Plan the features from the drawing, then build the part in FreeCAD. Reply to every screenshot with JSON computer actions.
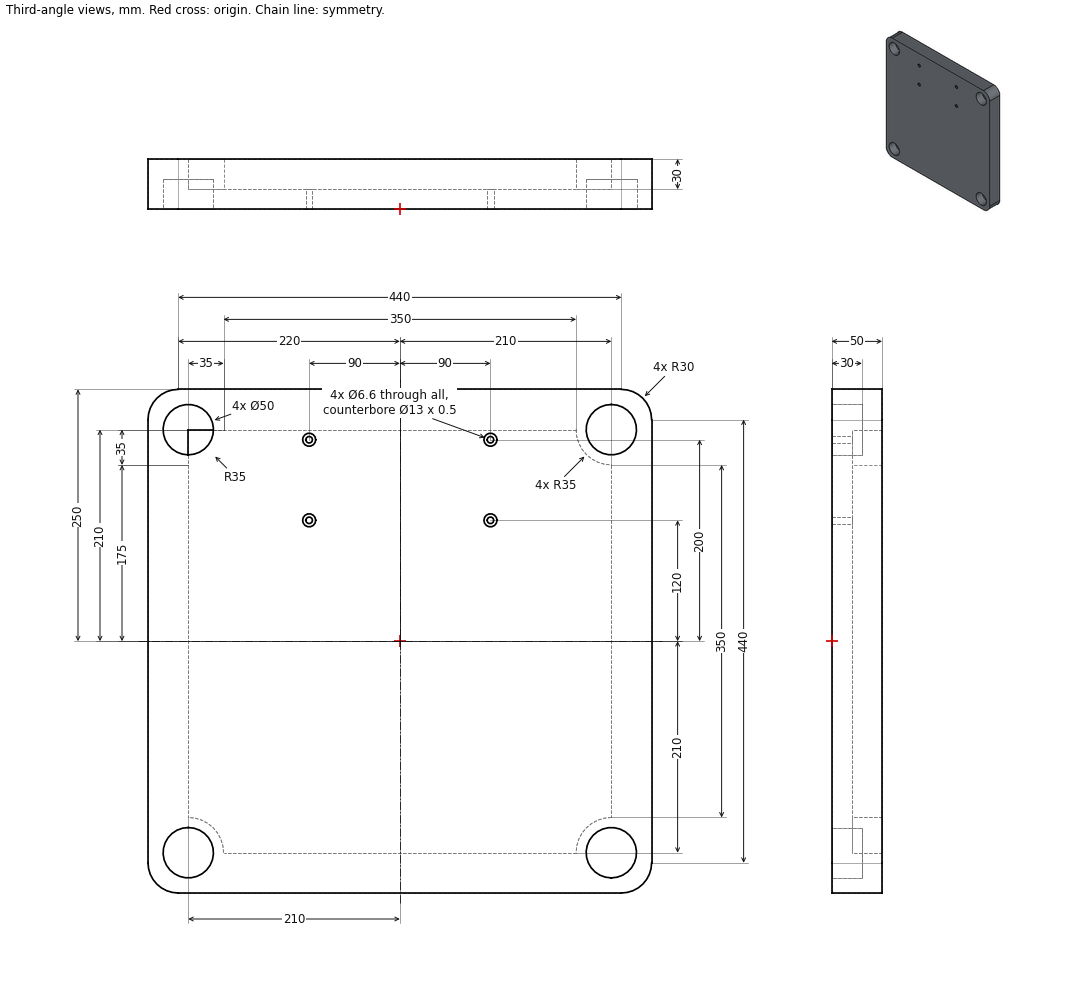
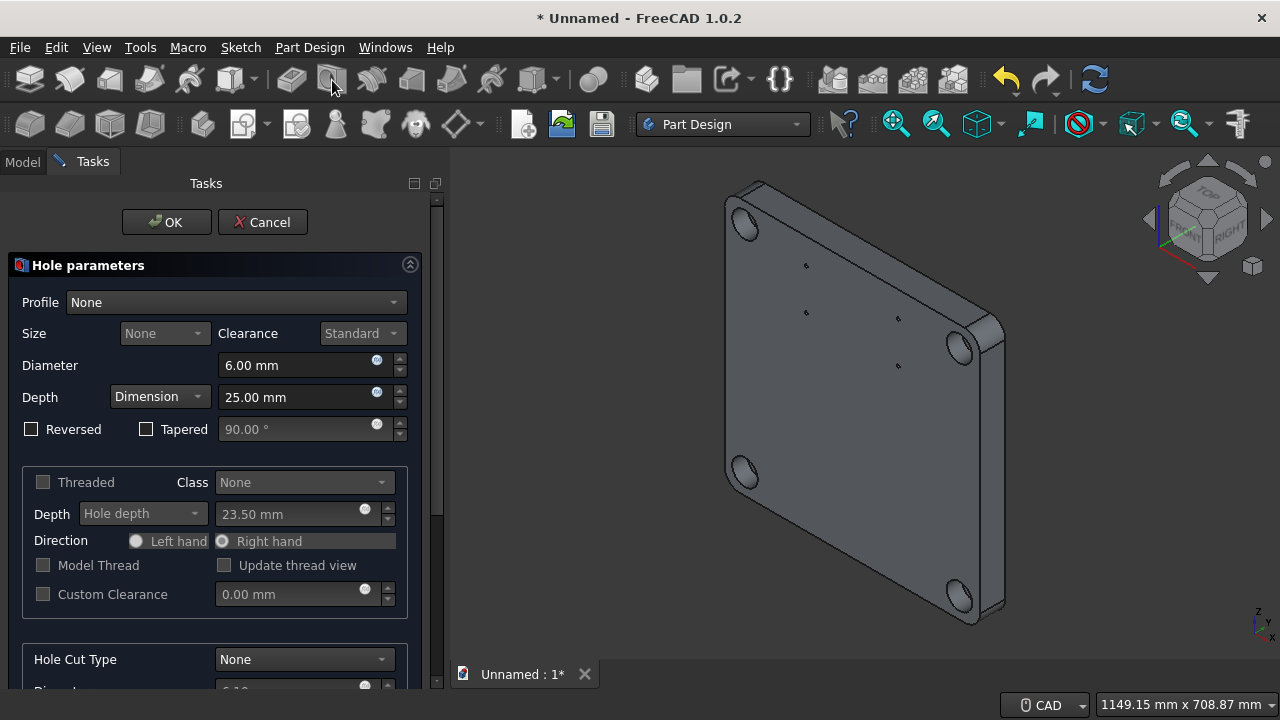
{"action": "triple_click", "coordinate": [305, 365]}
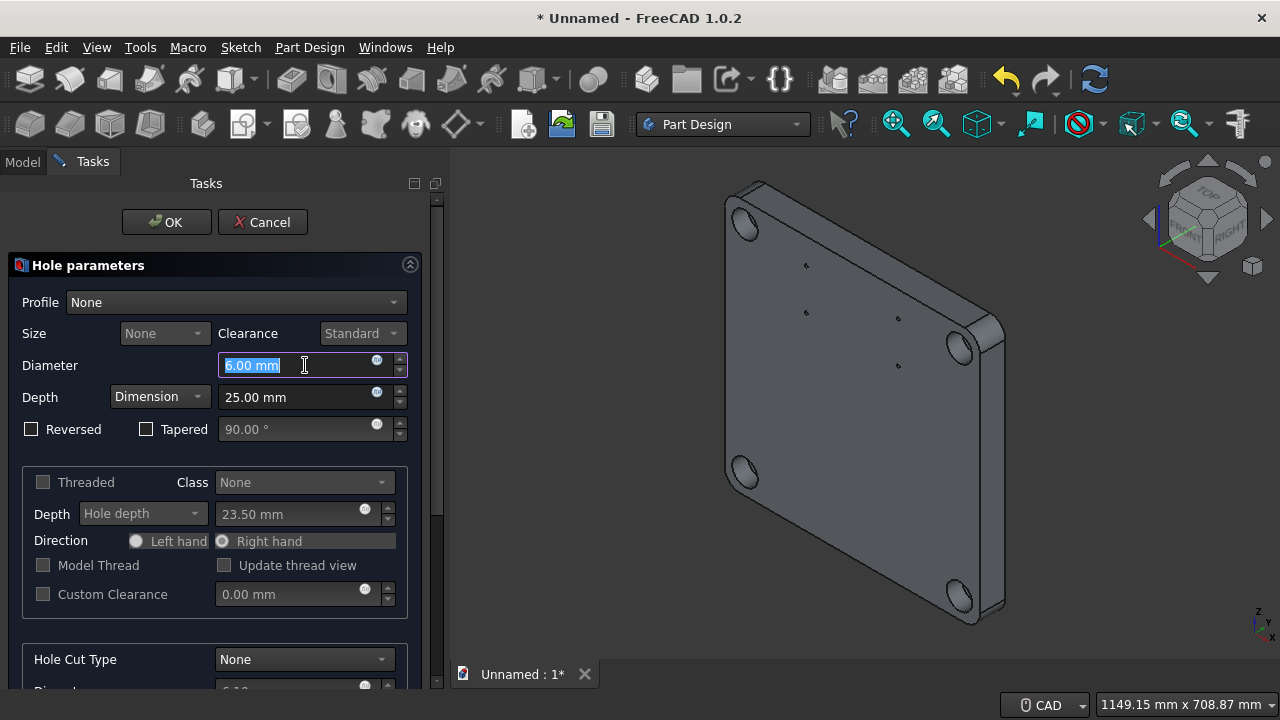
{"action": "type", "text": "6.6"}
{"action": "key", "text": "Tab"}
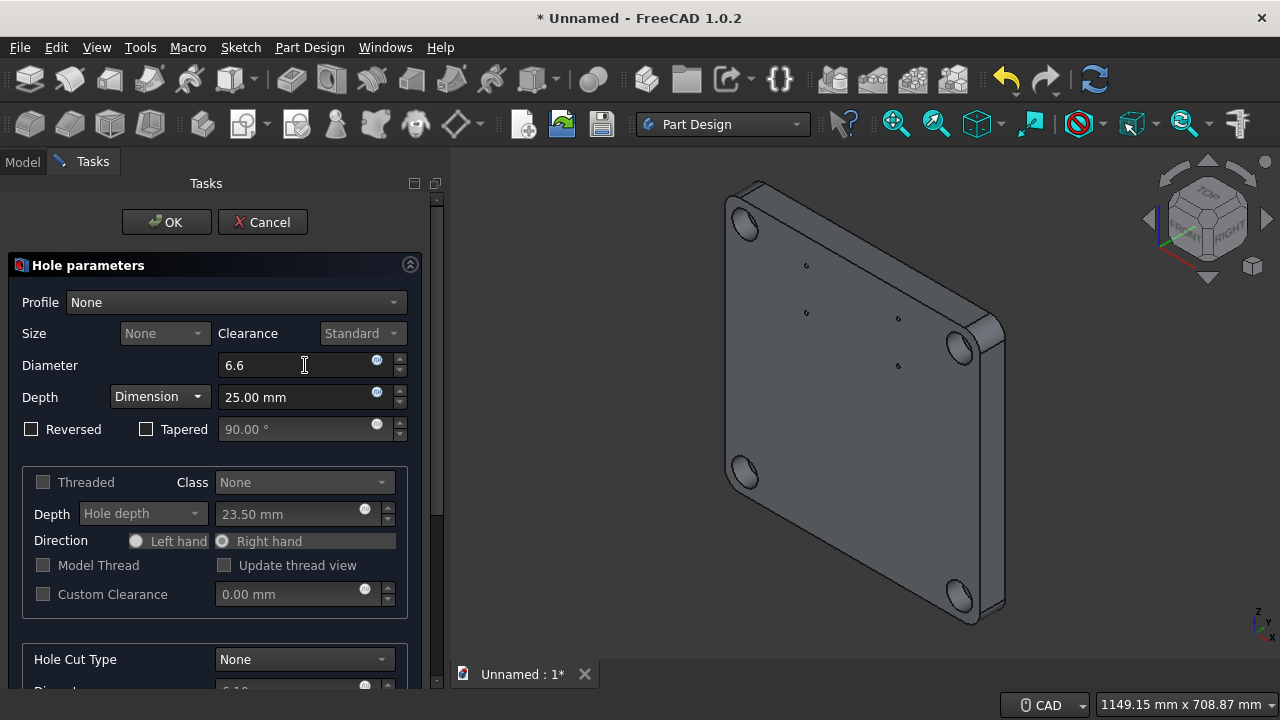
{"action": "left_click", "coordinate": [161, 396]}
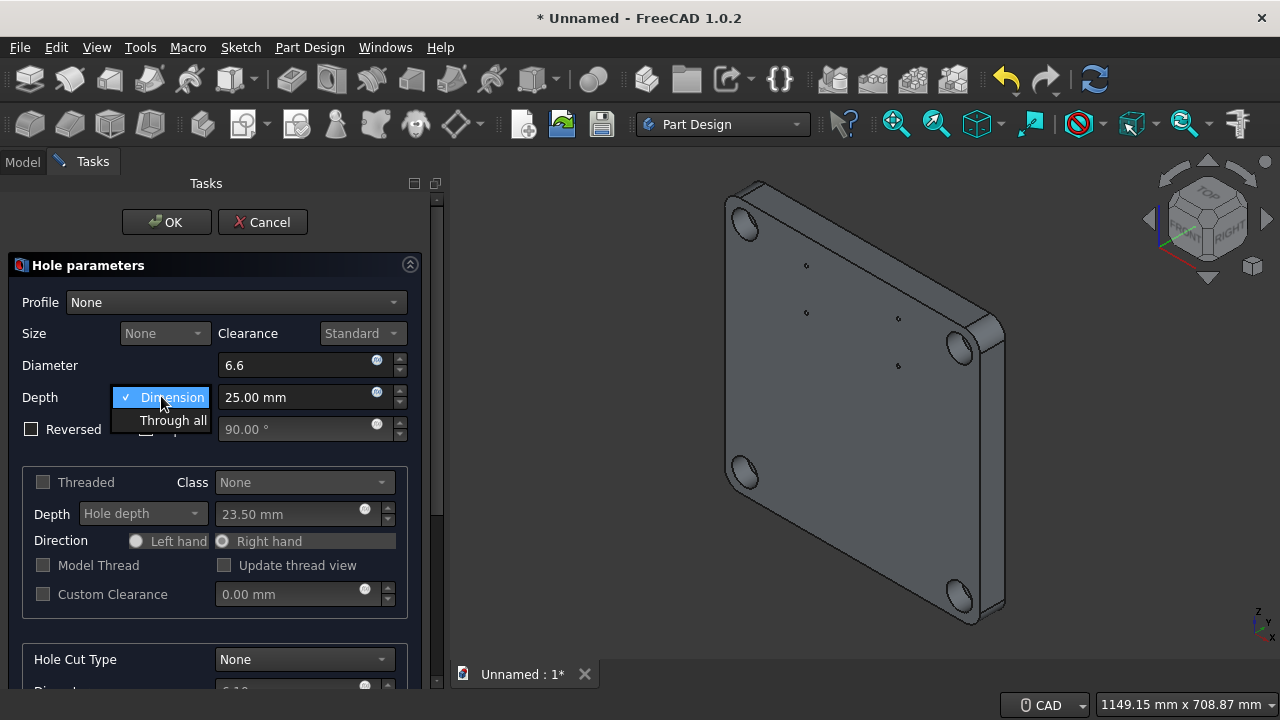
{"action": "left_click", "coordinate": [160, 420]}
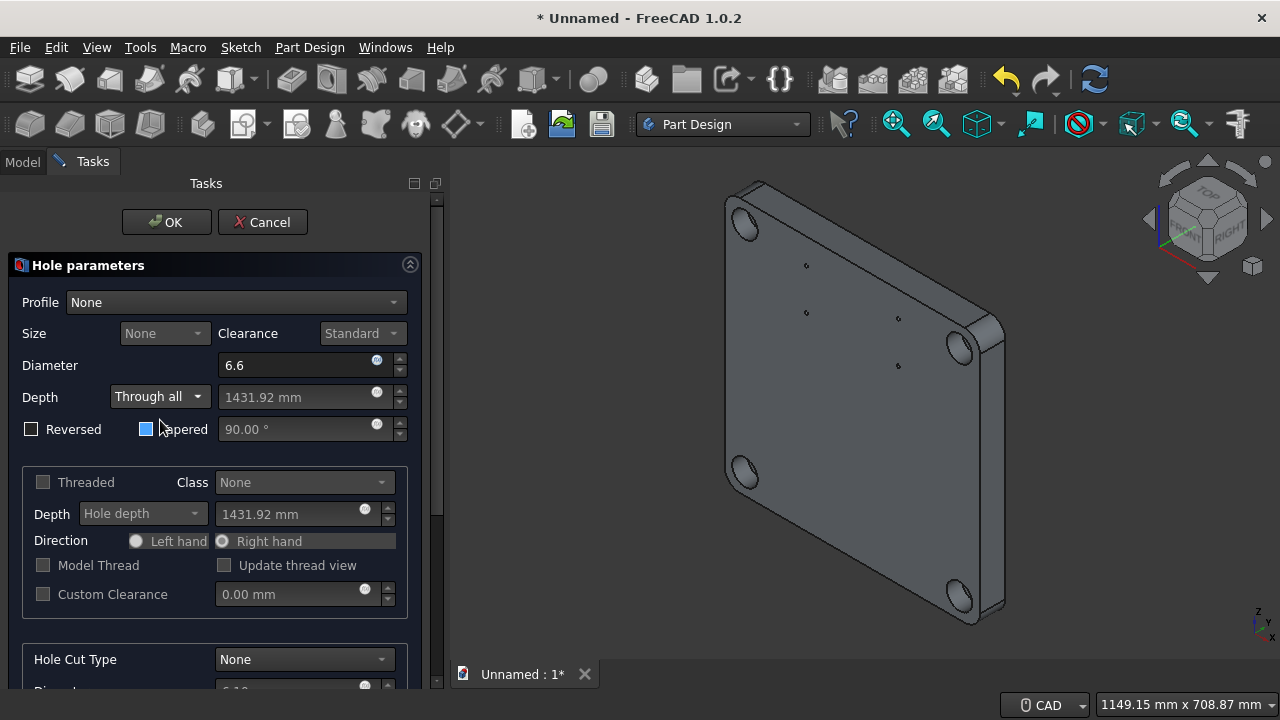
{"action": "left_click", "coordinate": [306, 660]}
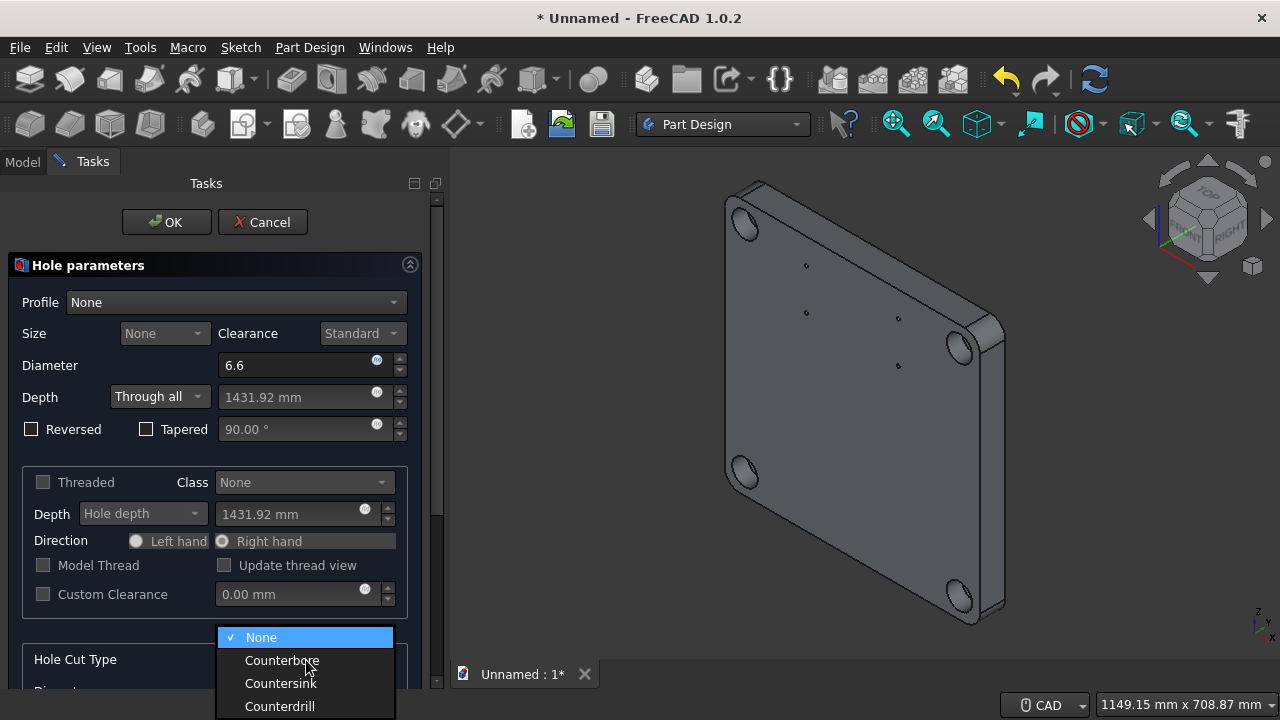
{"action": "left_click", "coordinate": [304, 660]}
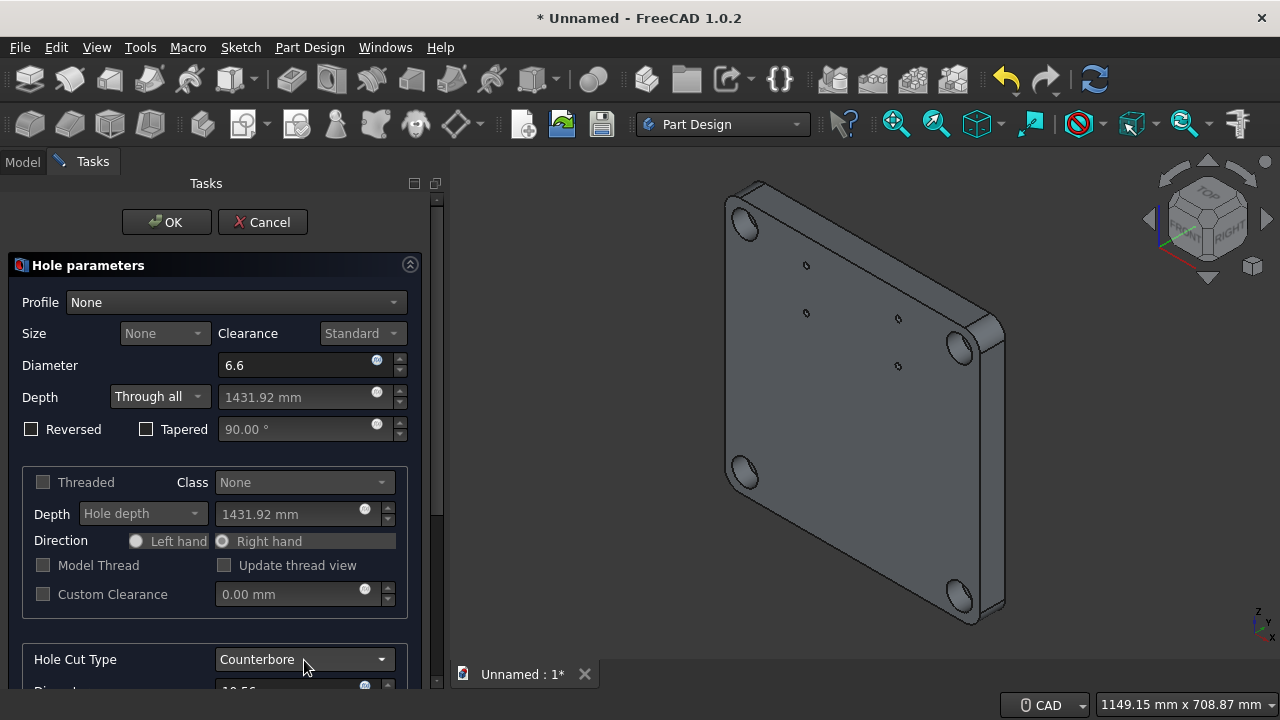
{"action": "scroll", "coordinate": [437, 440], "scroll_direction": "down", "scroll_amount": 2}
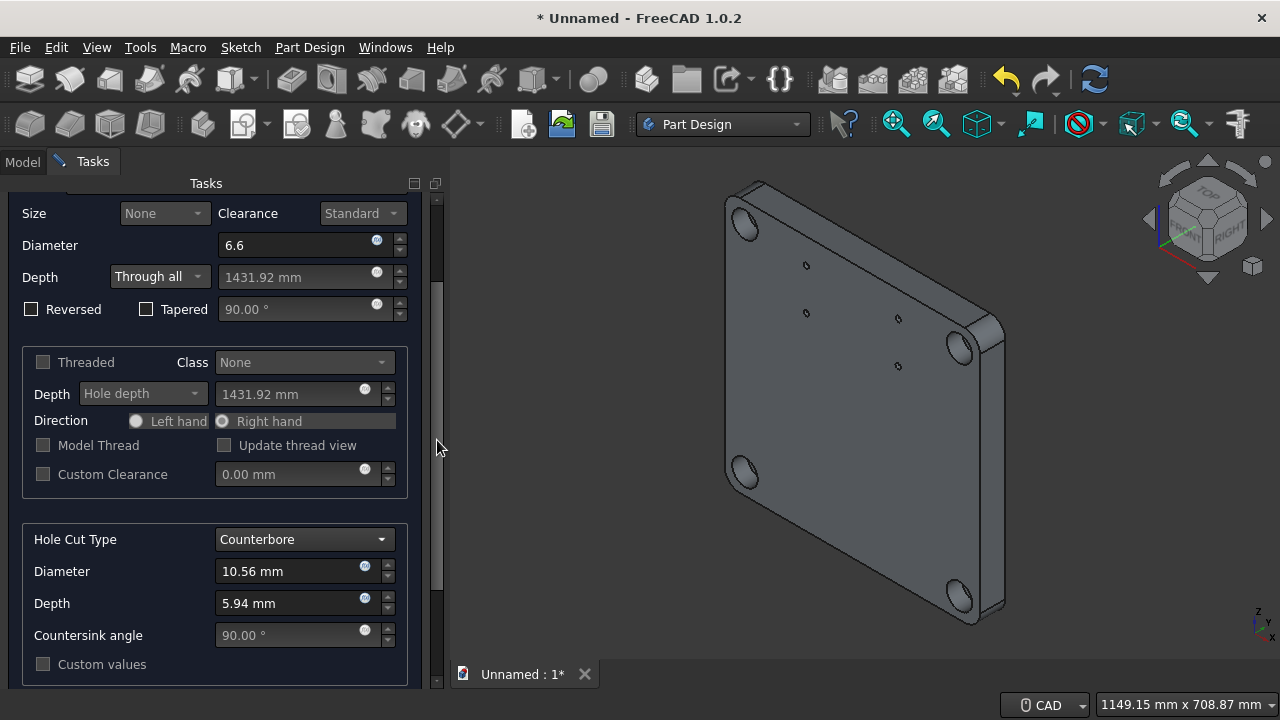
{"action": "triple_click", "coordinate": [298, 571]}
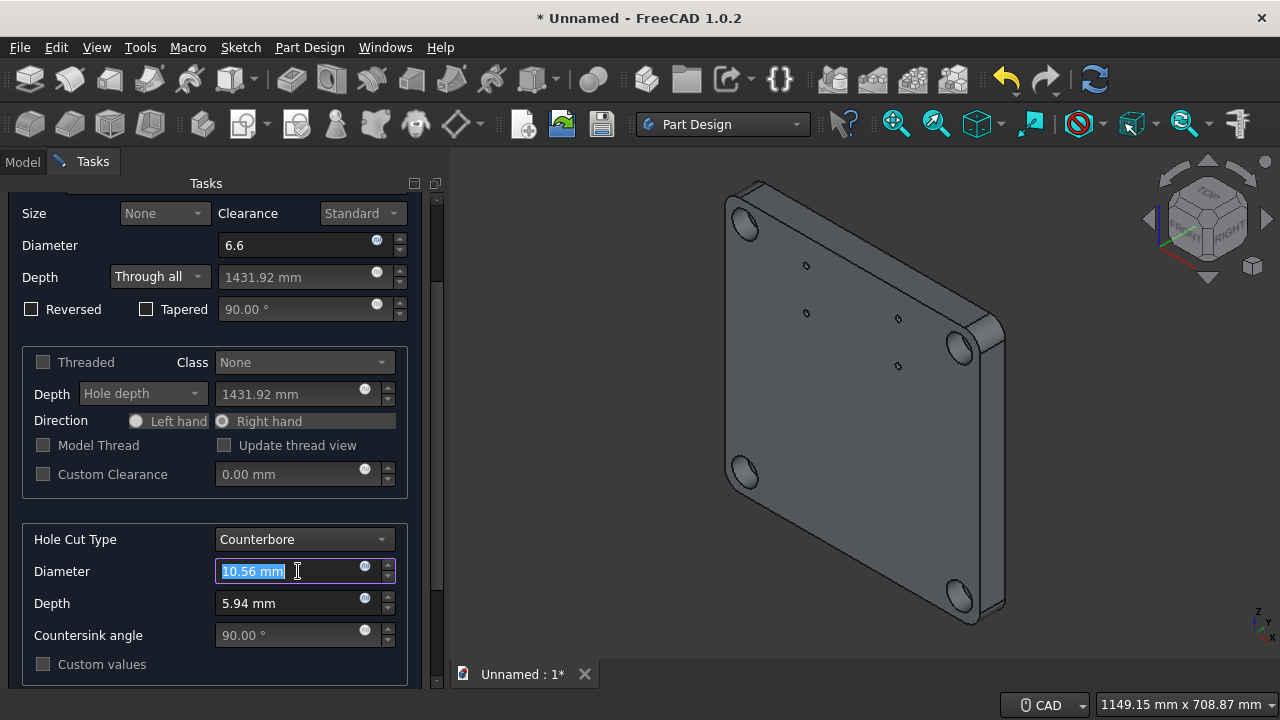
{"action": "type", "text": "13"}
{"action": "key", "text": "Tab"}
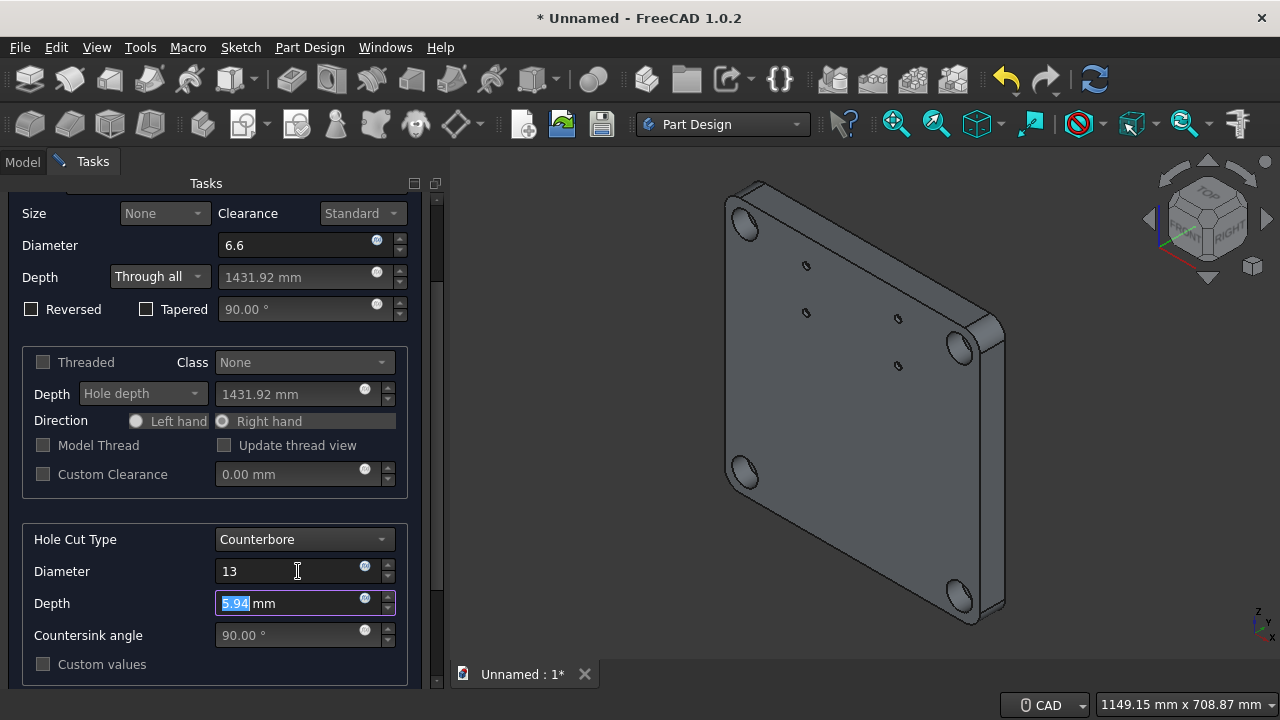
{"action": "type", "text": "0.5"}
{"action": "key", "text": "Tab"}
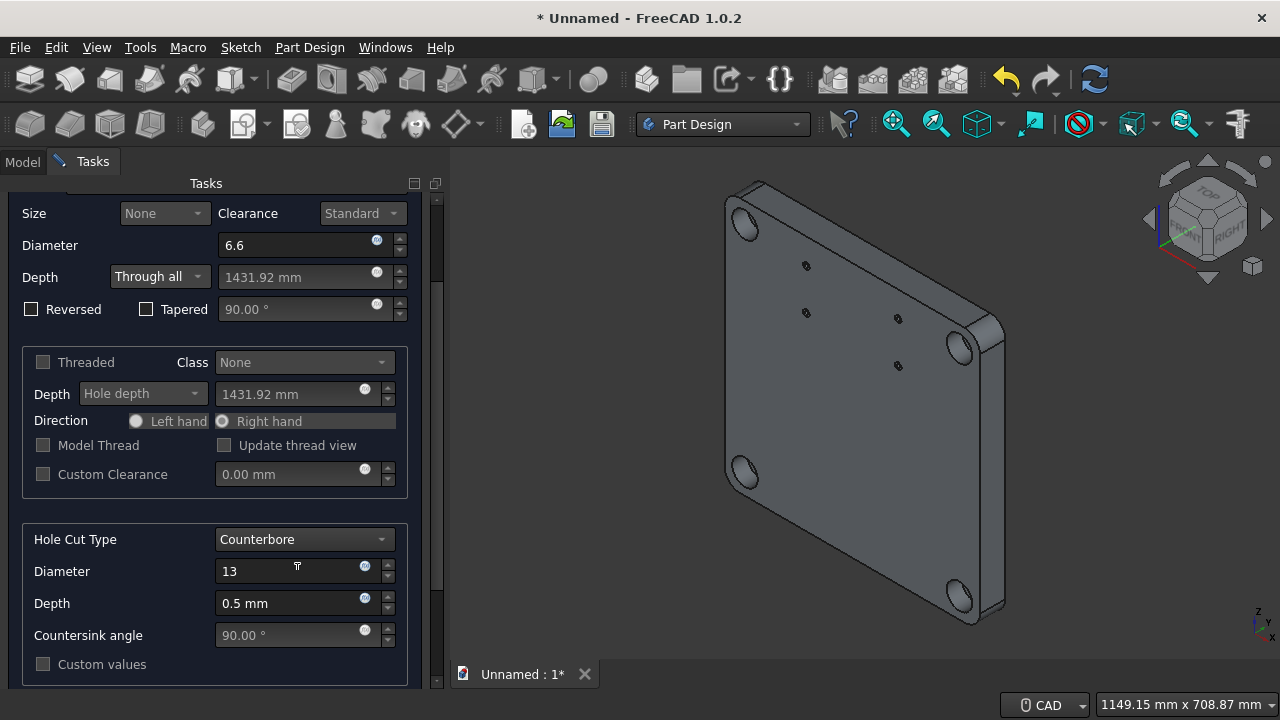
{"action": "scroll", "coordinate": [437, 440], "scroll_direction": "up", "scroll_amount": 3}